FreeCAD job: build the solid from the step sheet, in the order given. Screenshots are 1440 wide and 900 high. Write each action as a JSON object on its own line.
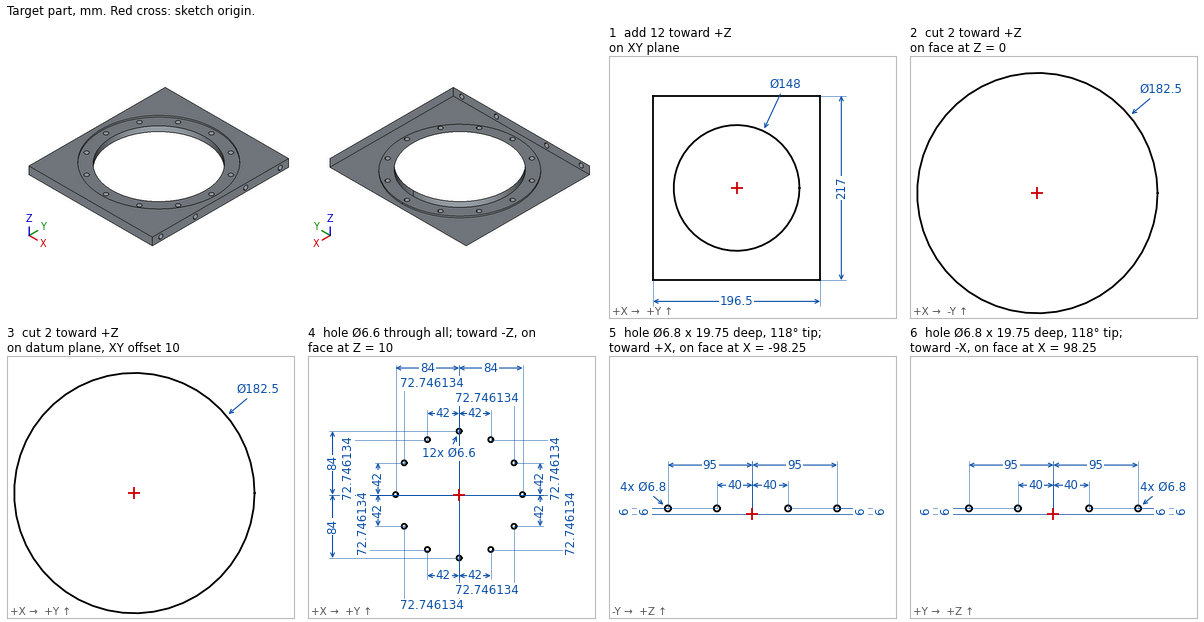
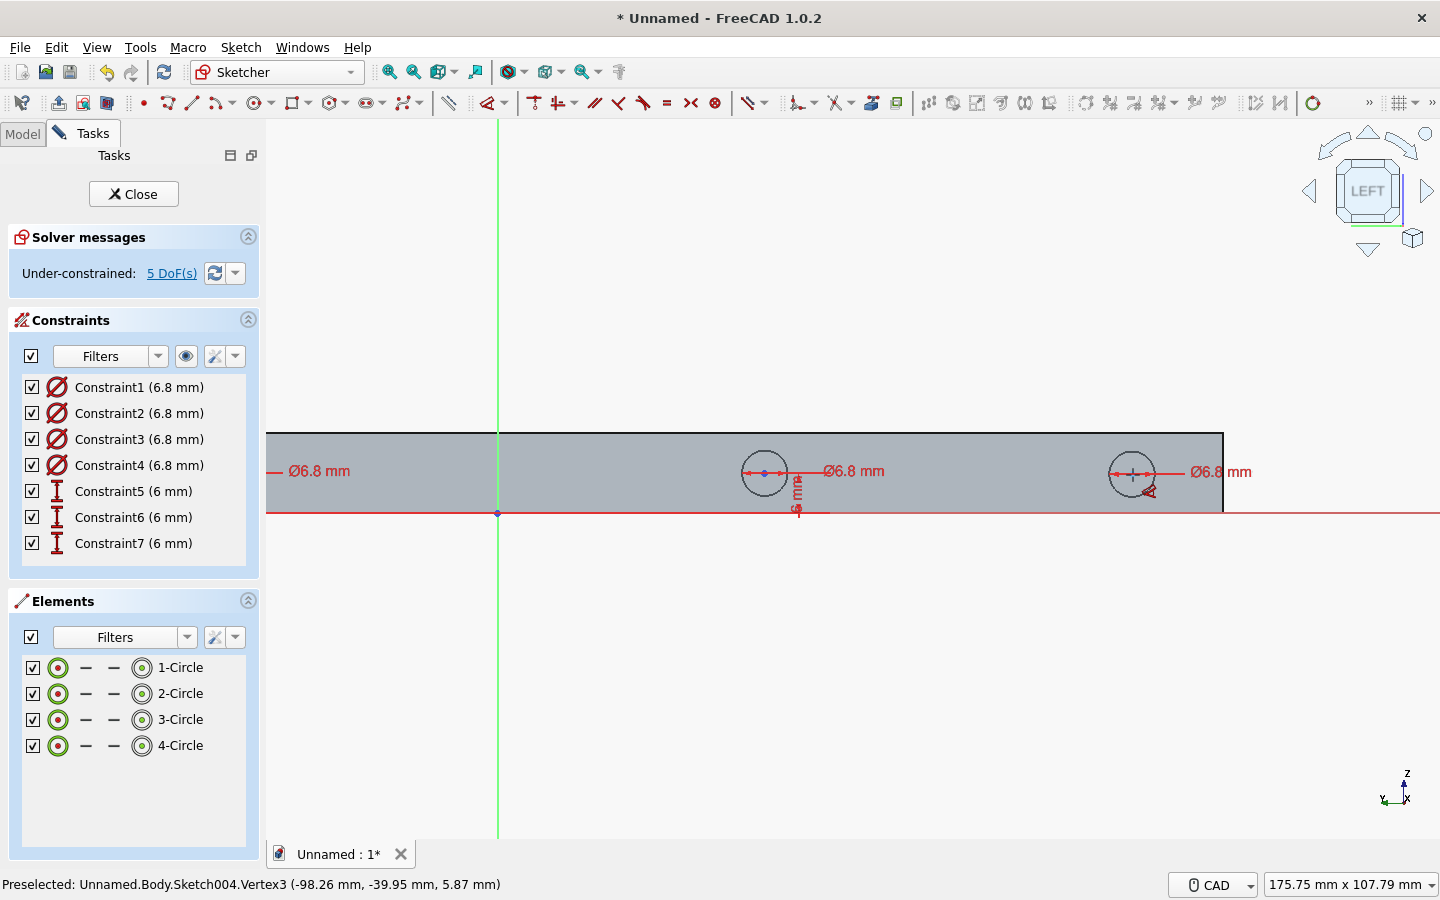
{"action": "left_click", "coordinate": [1132, 474]}
{"action": "left_click", "coordinate": [1166, 494]}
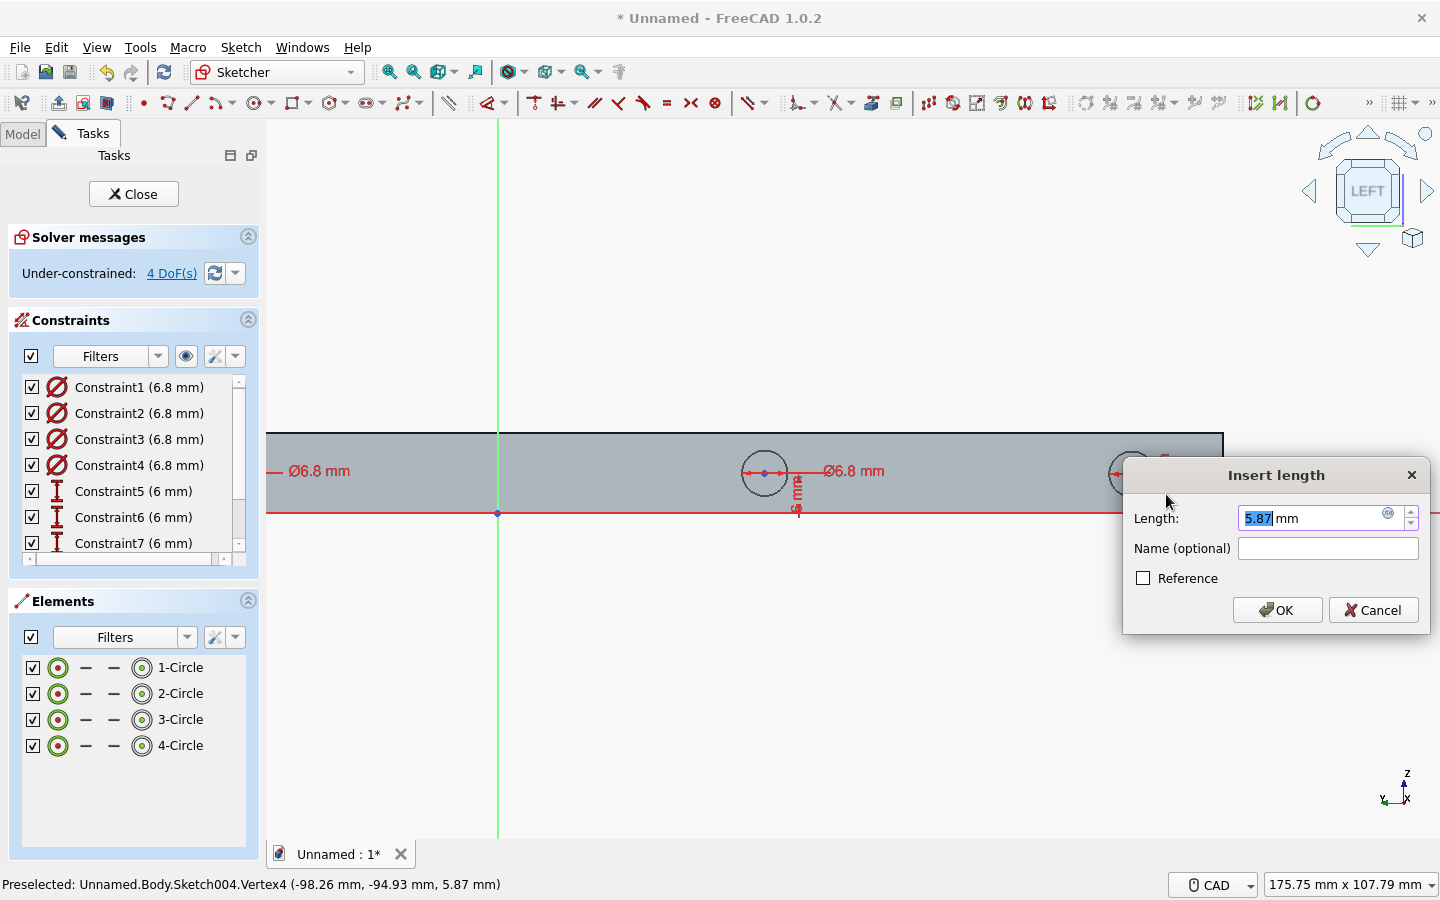
{"action": "type", "text": "6"}
{"action": "key", "text": "Return"}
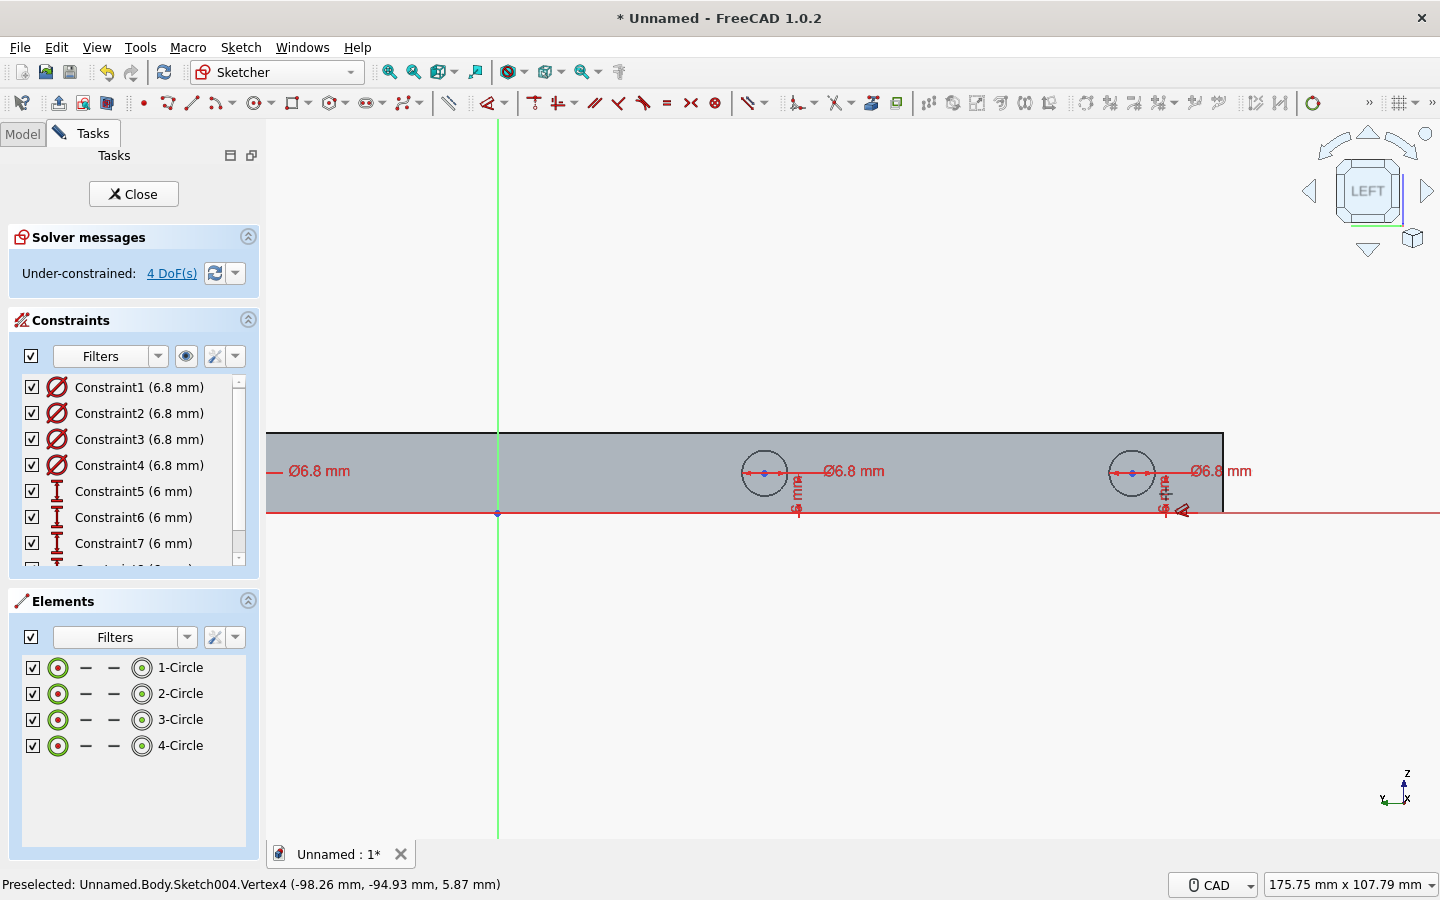
{"action": "scroll", "coordinate": [1133, 475], "scroll_direction": "down", "scroll_amount": 3}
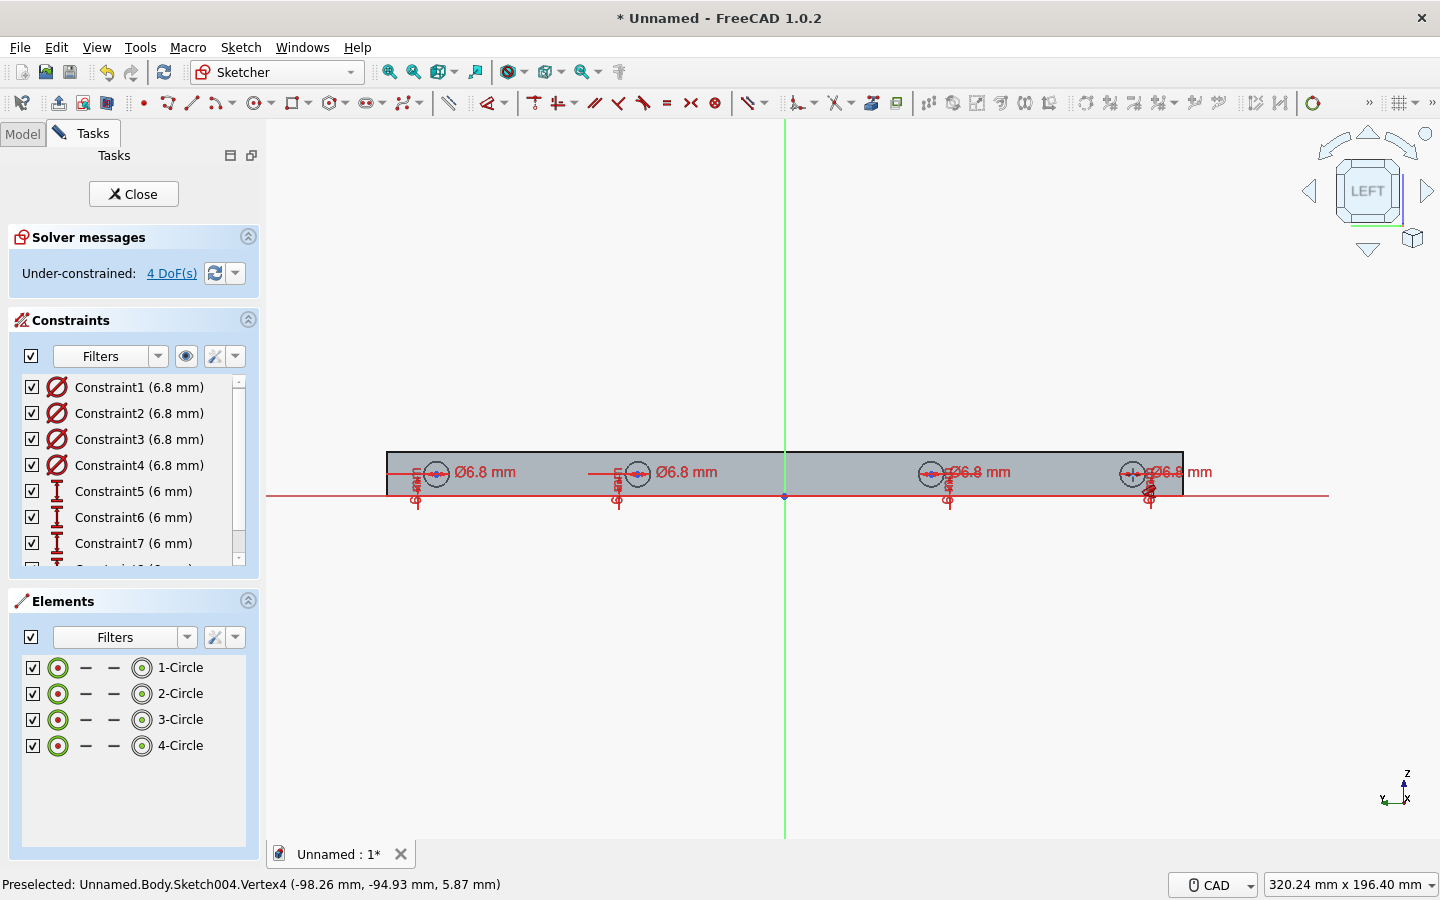
{"action": "left_click", "coordinate": [437, 474]}
{"action": "left_click", "coordinate": [611, 530]}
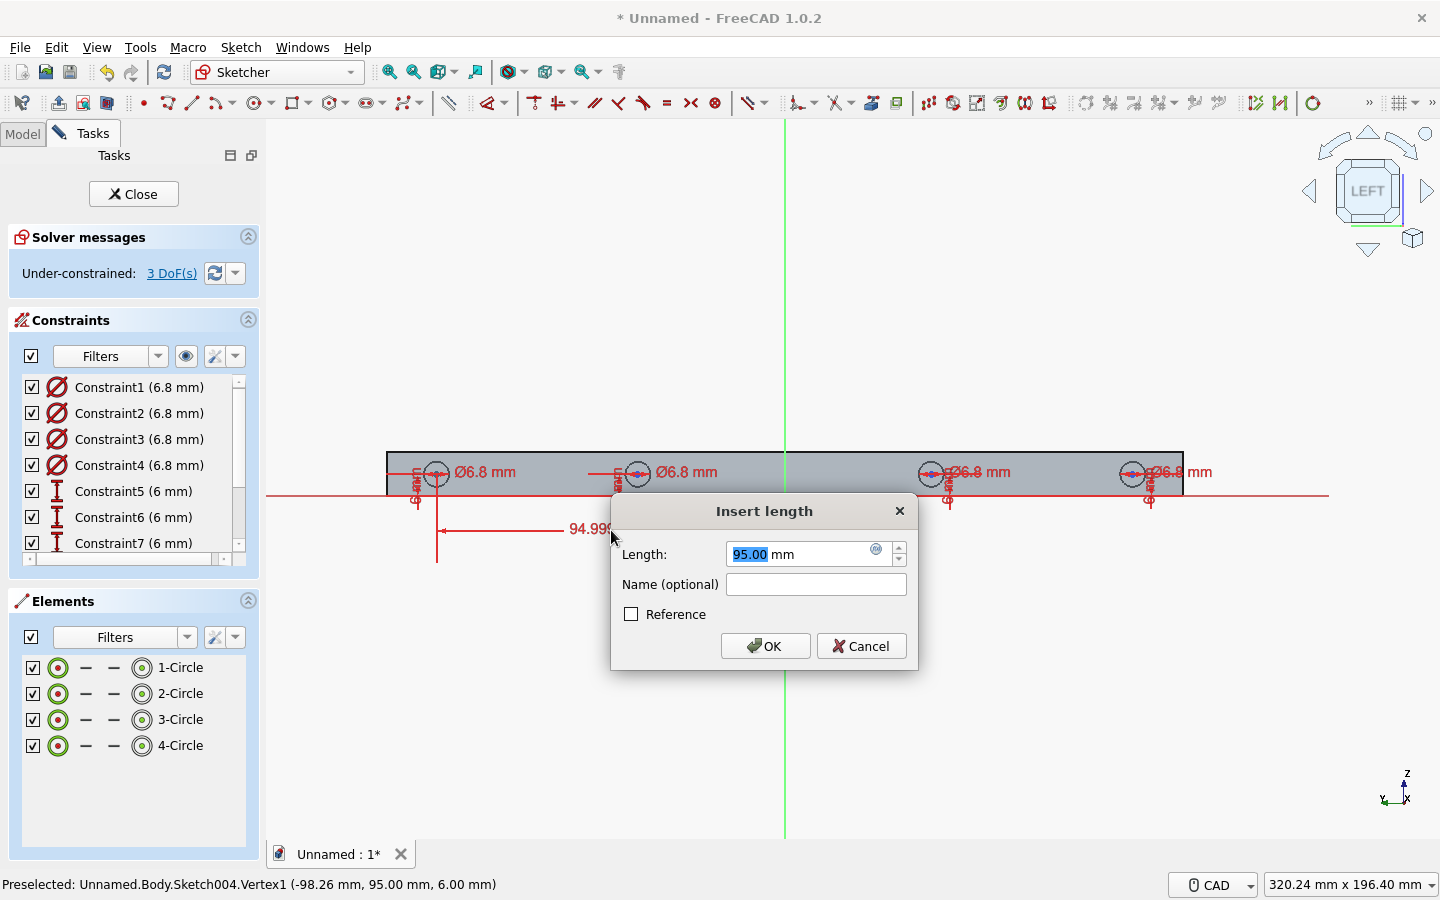
{"action": "type", "text": "95"}
{"action": "key", "text": "Return"}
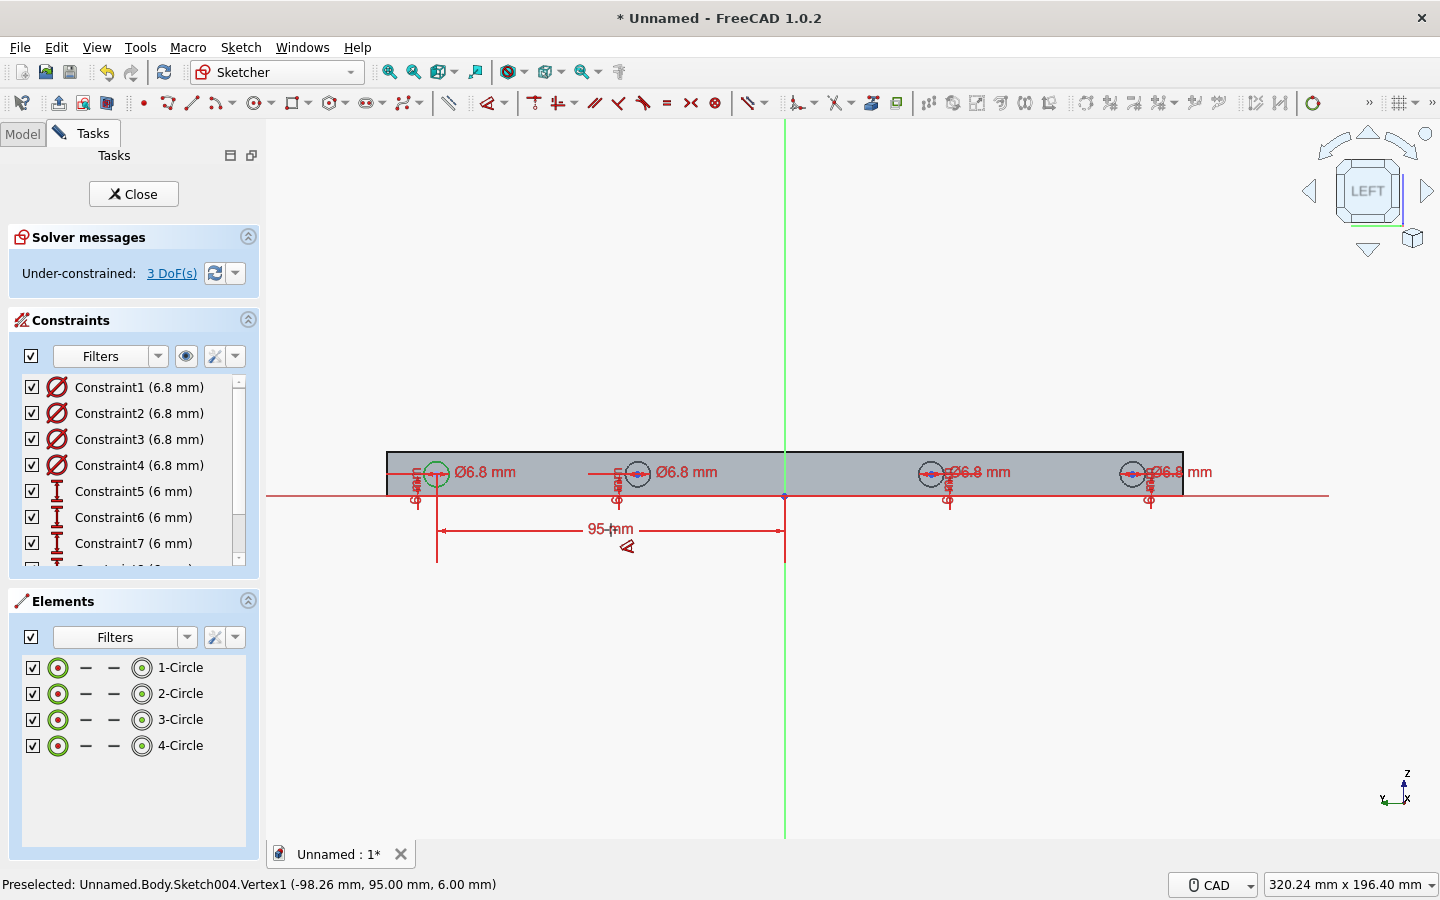
{"action": "left_click", "coordinate": [638, 474]}
{"action": "left_click", "coordinate": [711, 530]}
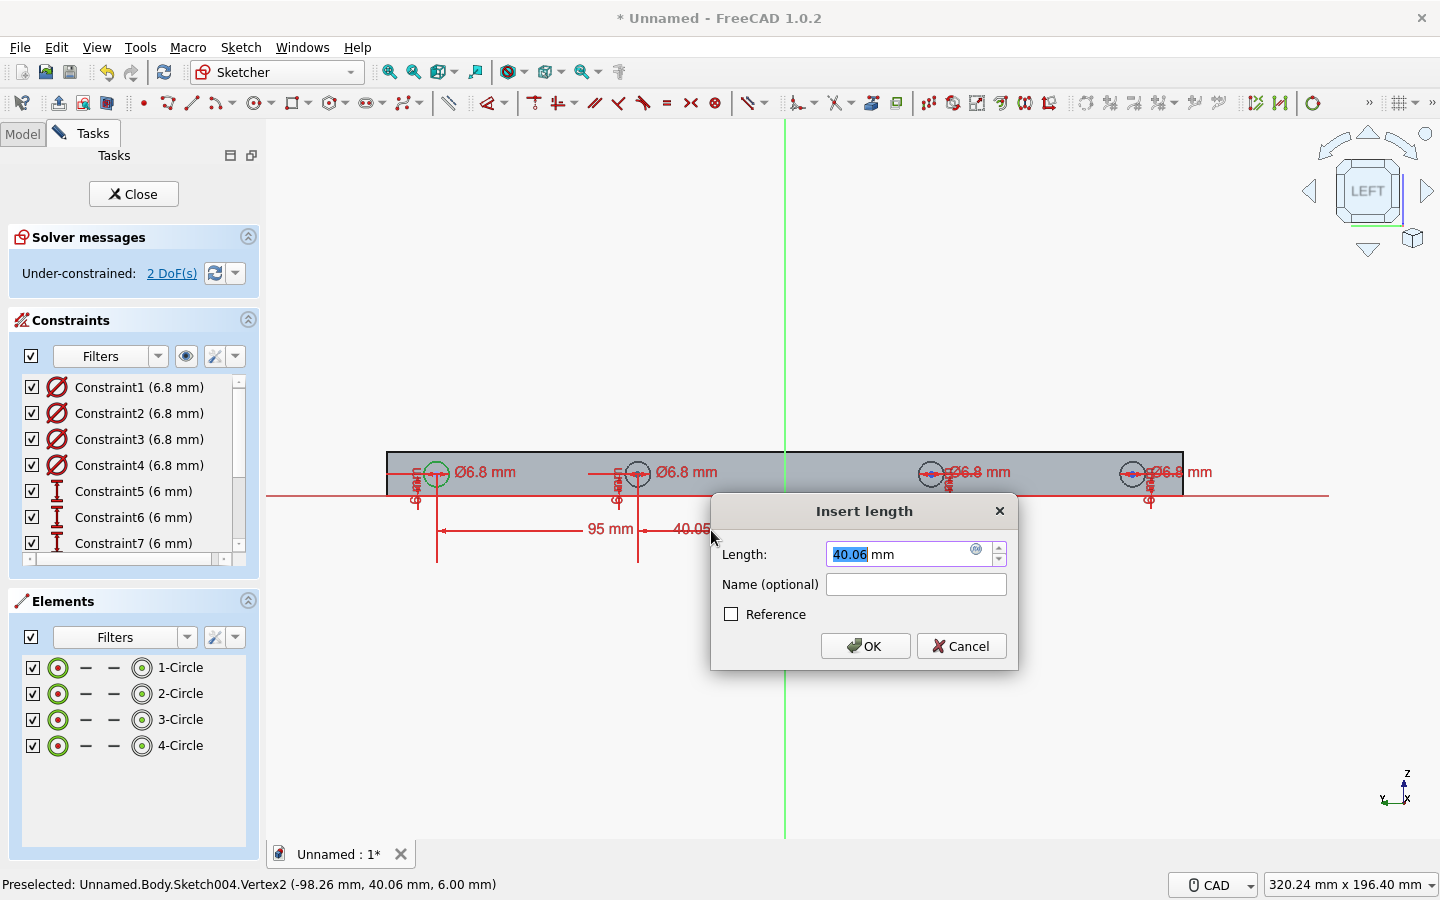
{"action": "type", "text": "40"}
{"action": "key", "text": "Return"}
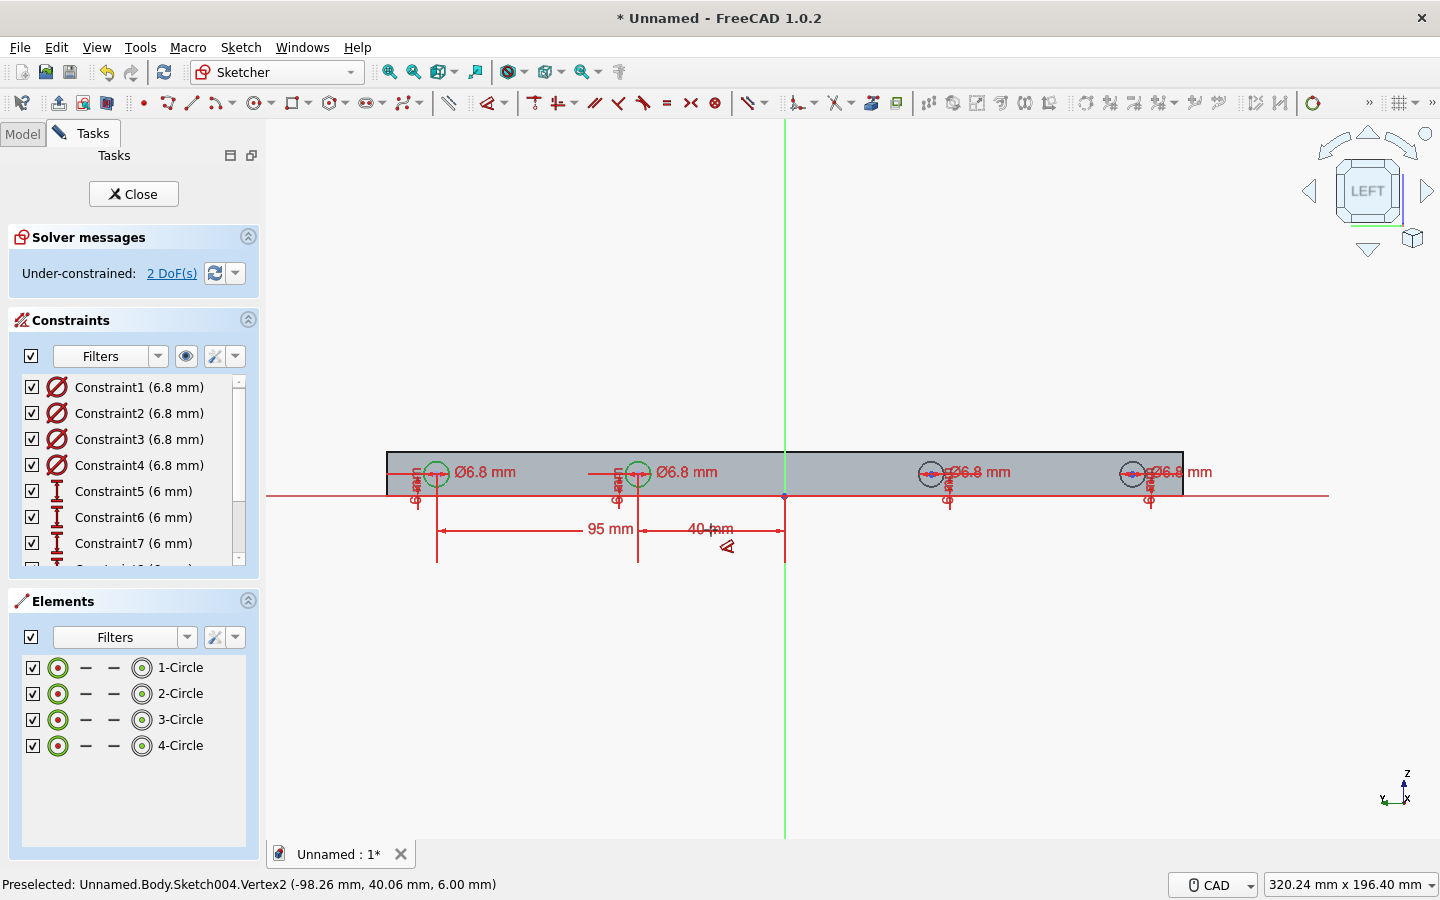
{"action": "left_click", "coordinate": [931, 474]}
{"action": "left_click", "coordinate": [858, 530]}